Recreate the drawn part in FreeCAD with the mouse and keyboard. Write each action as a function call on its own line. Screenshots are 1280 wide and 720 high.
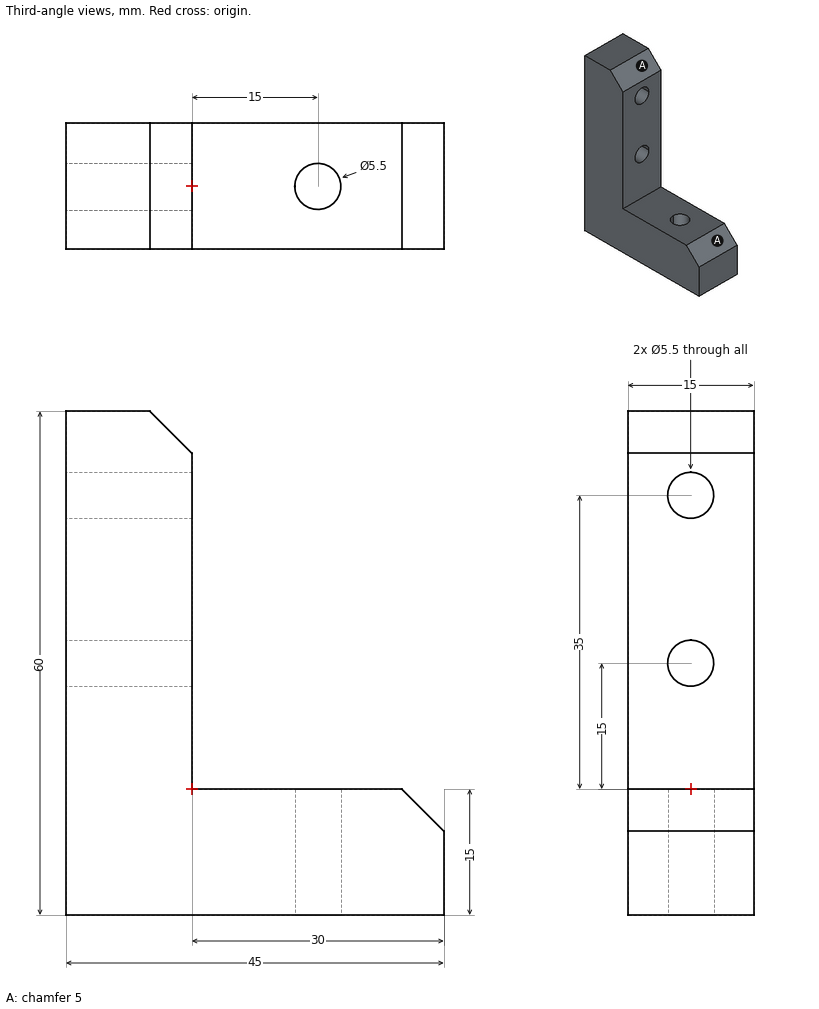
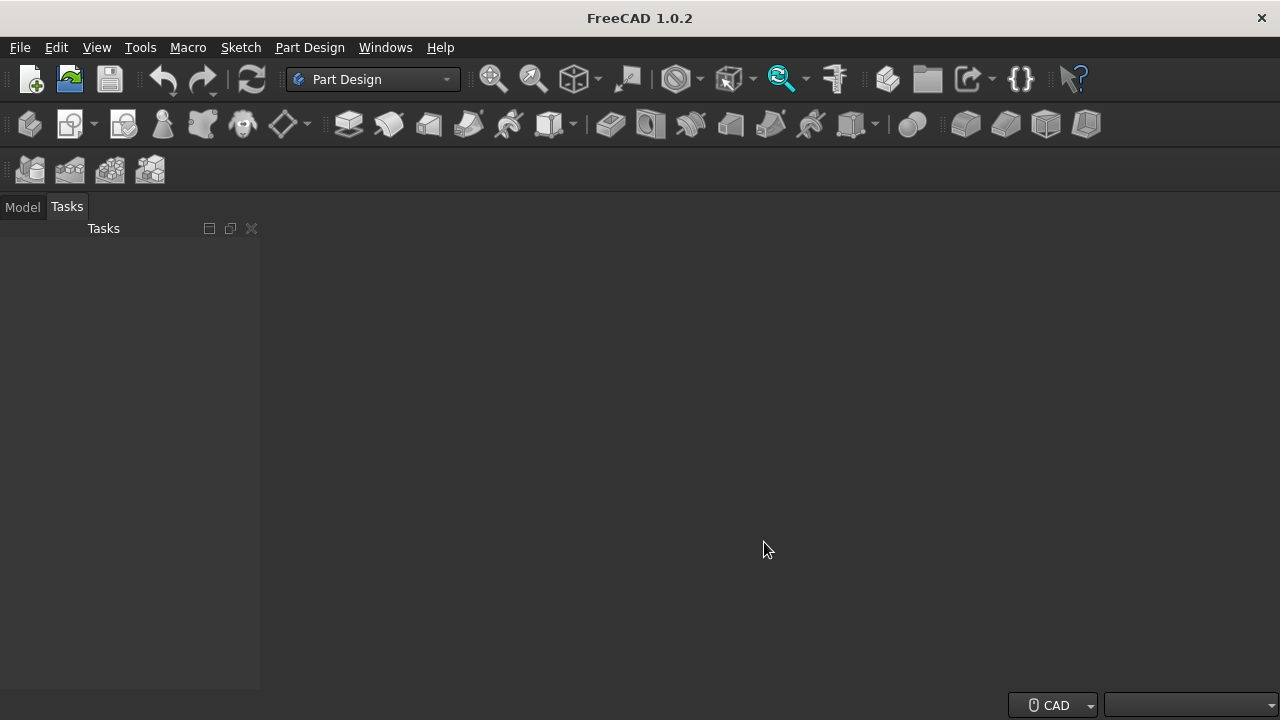
key(ctrl+n)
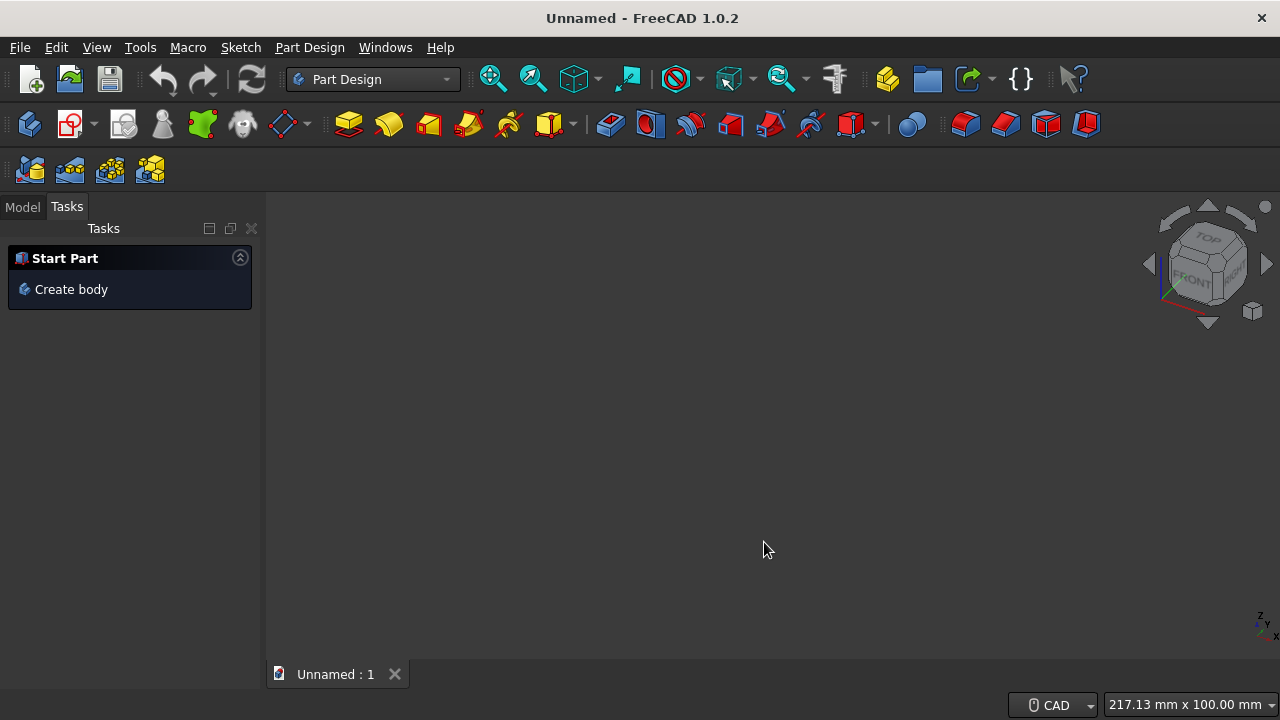
click(70, 124)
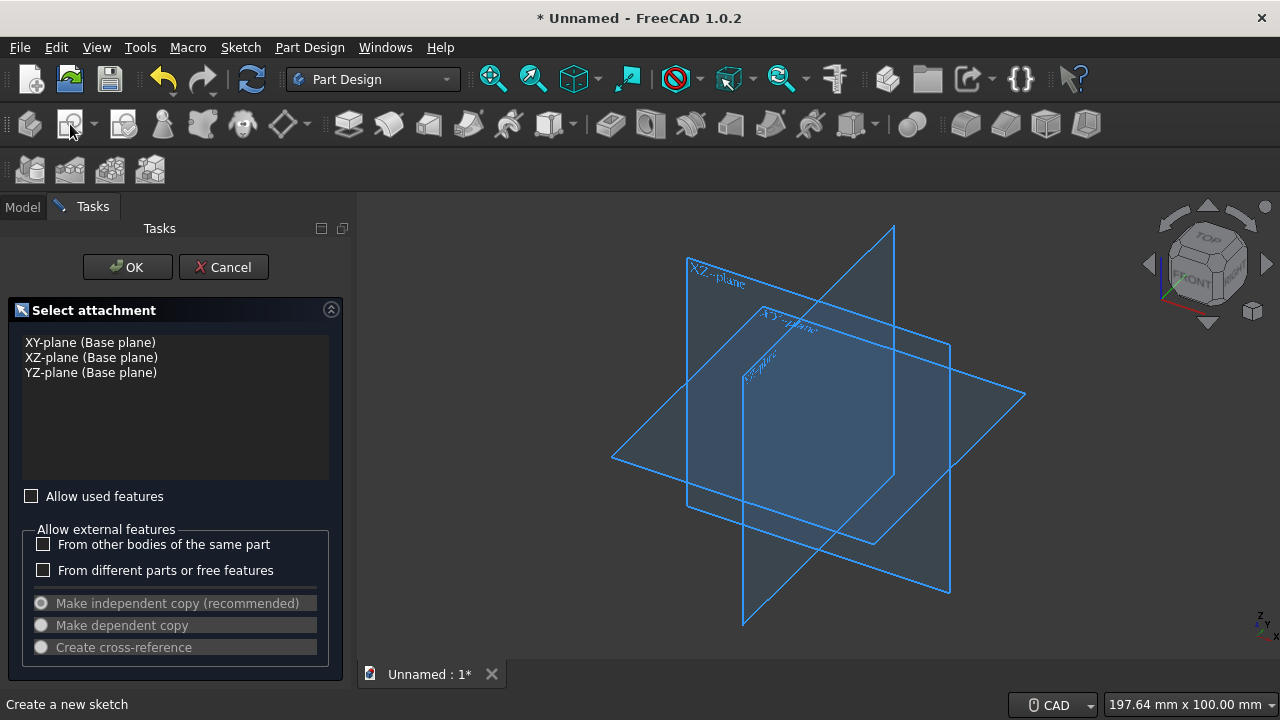
click(82, 358)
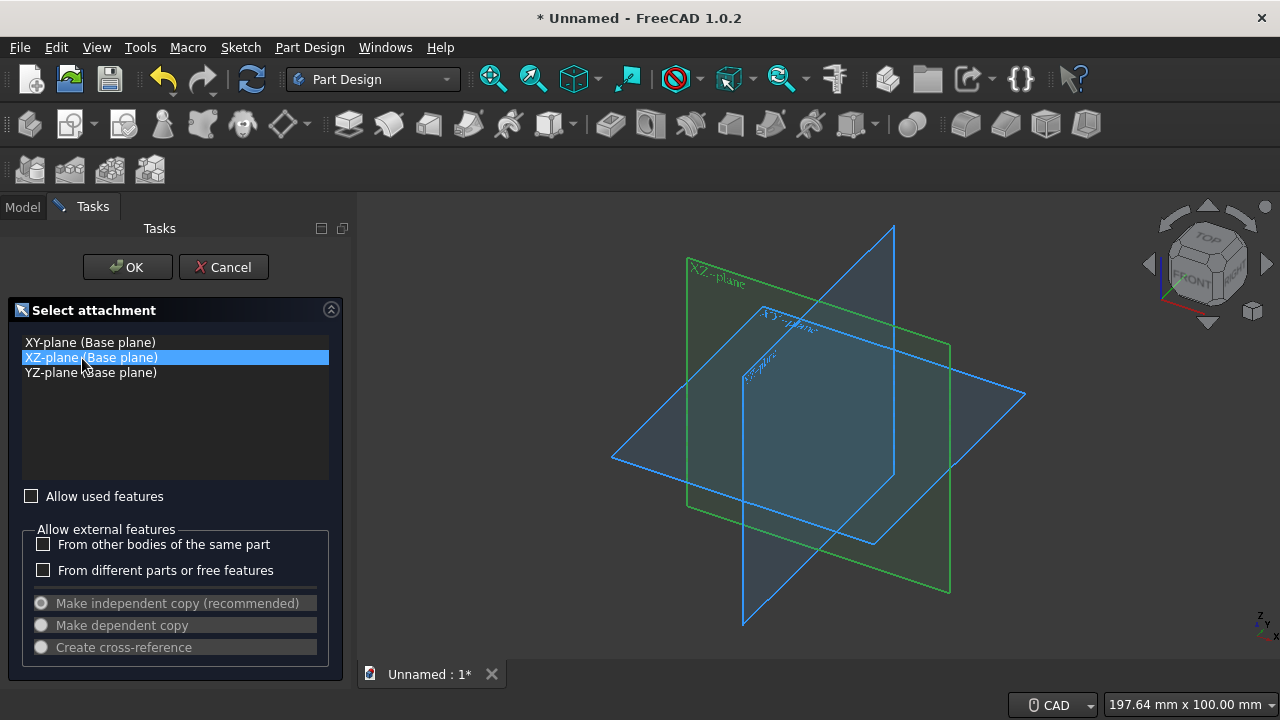
click(128, 267)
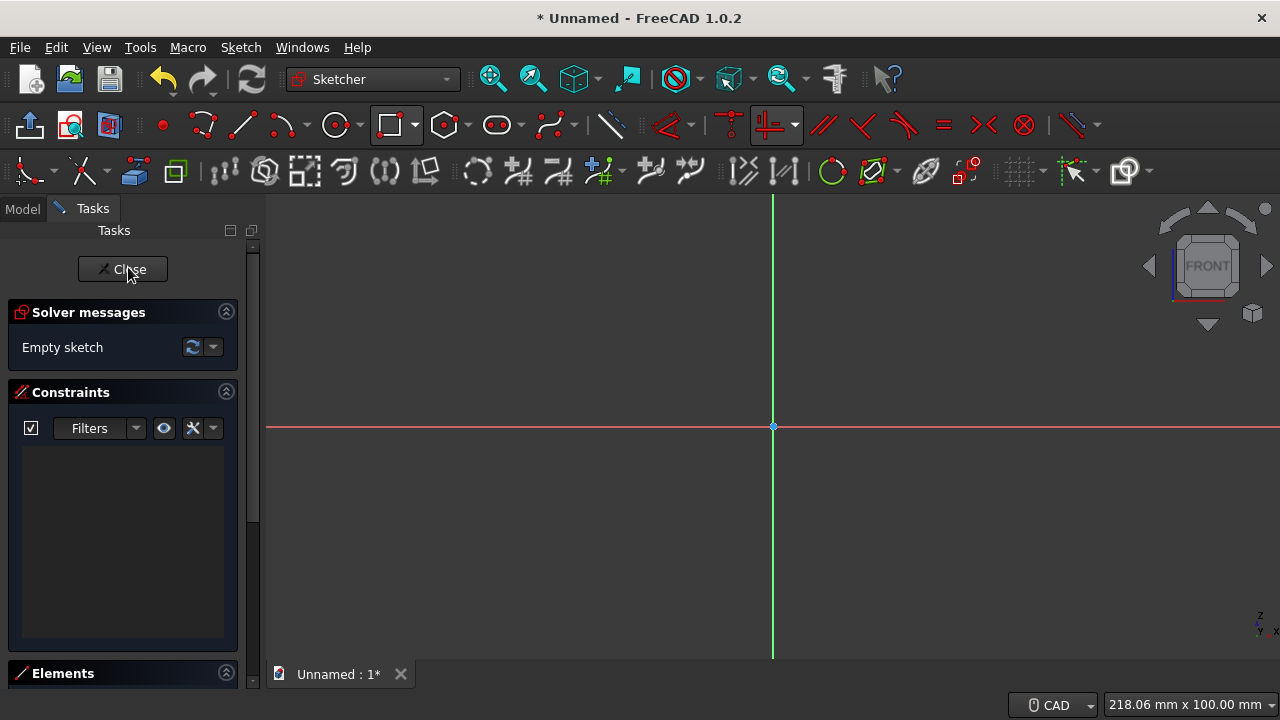
scroll(294, 631, down, 1)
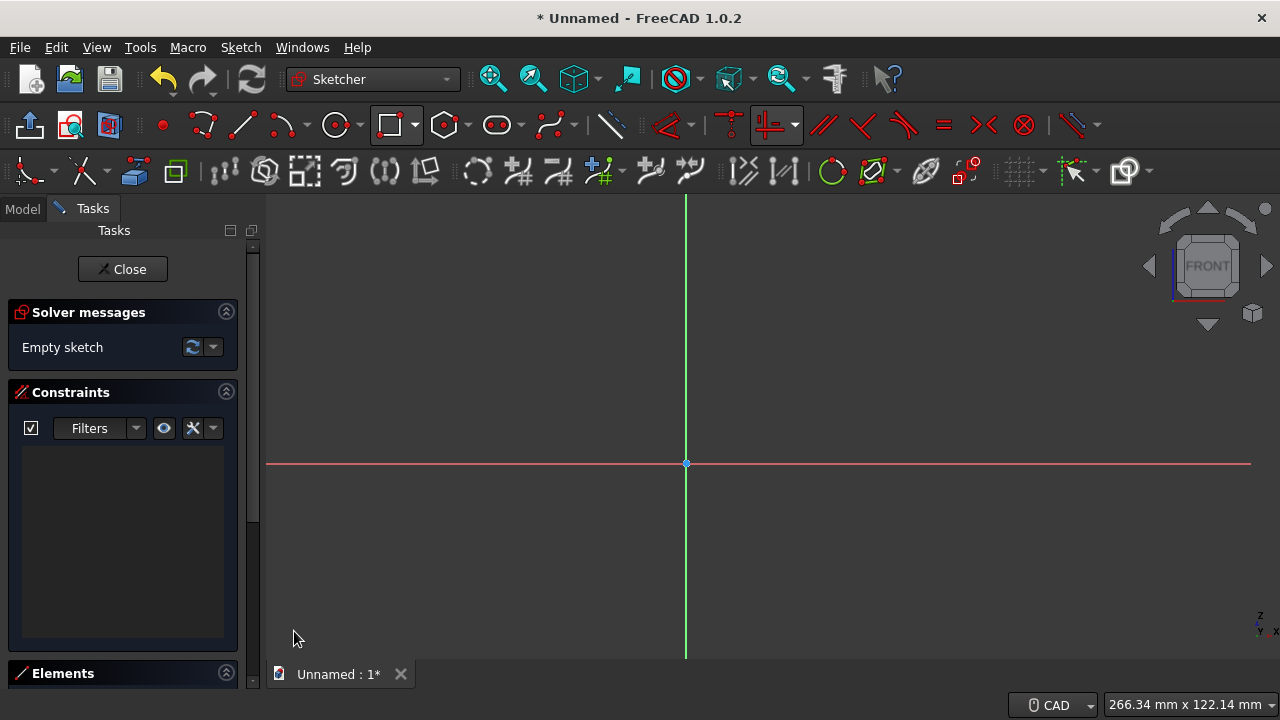
key(g)
key(m)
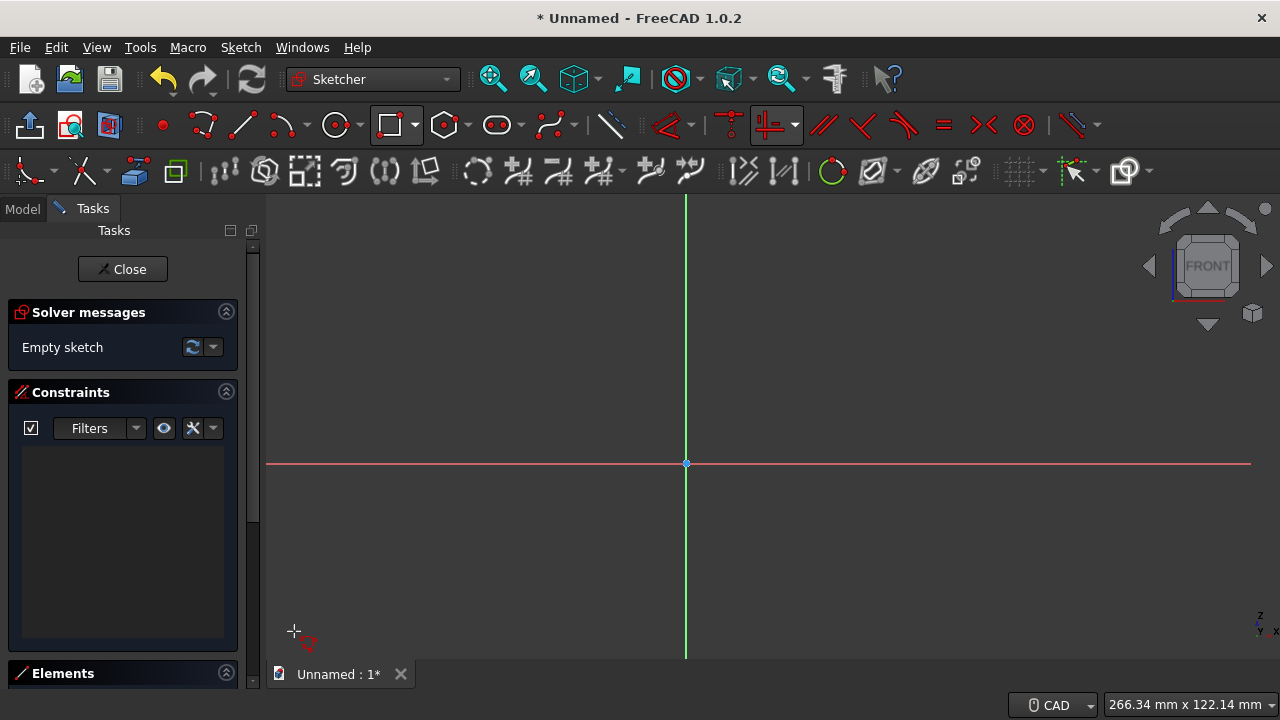
click(686, 464)
click(800, 455)
click(800, 521)
click(629, 521)
click(629, 292)
click(695, 292)
click(686, 464)
key(Escape)
key(Escape)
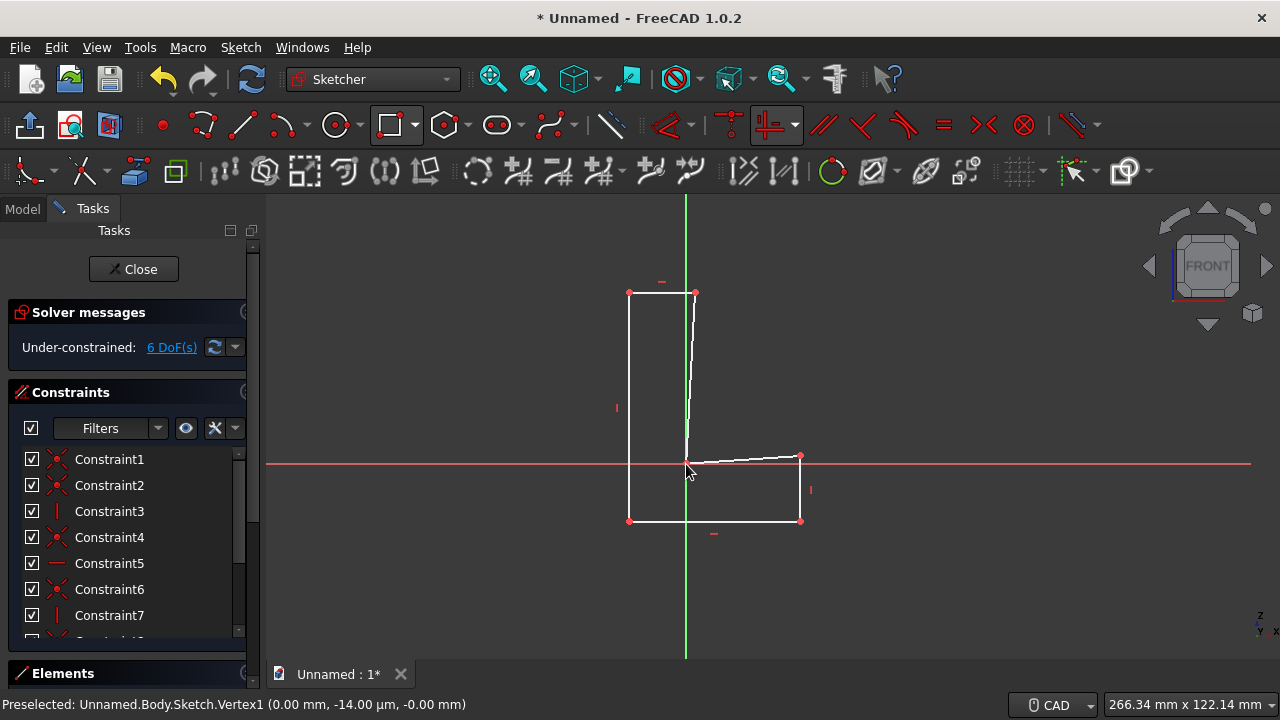
click(720, 461)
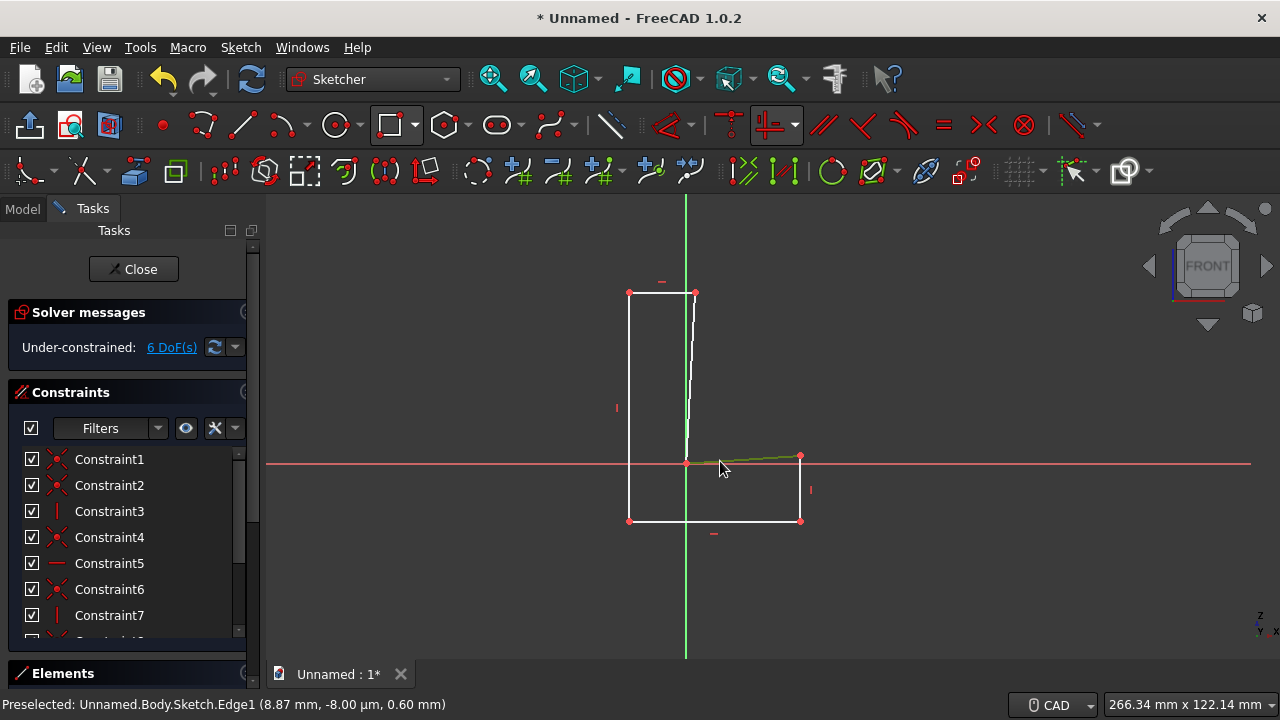
click(798, 126)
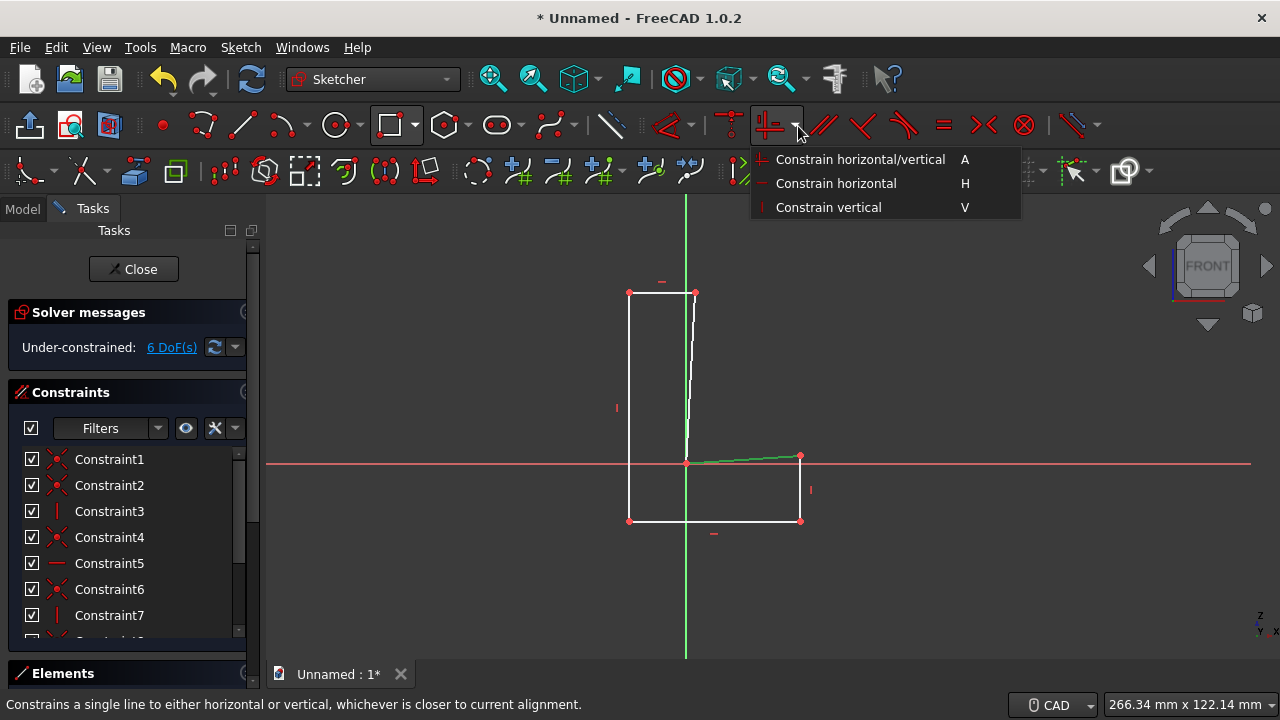
click(886, 183)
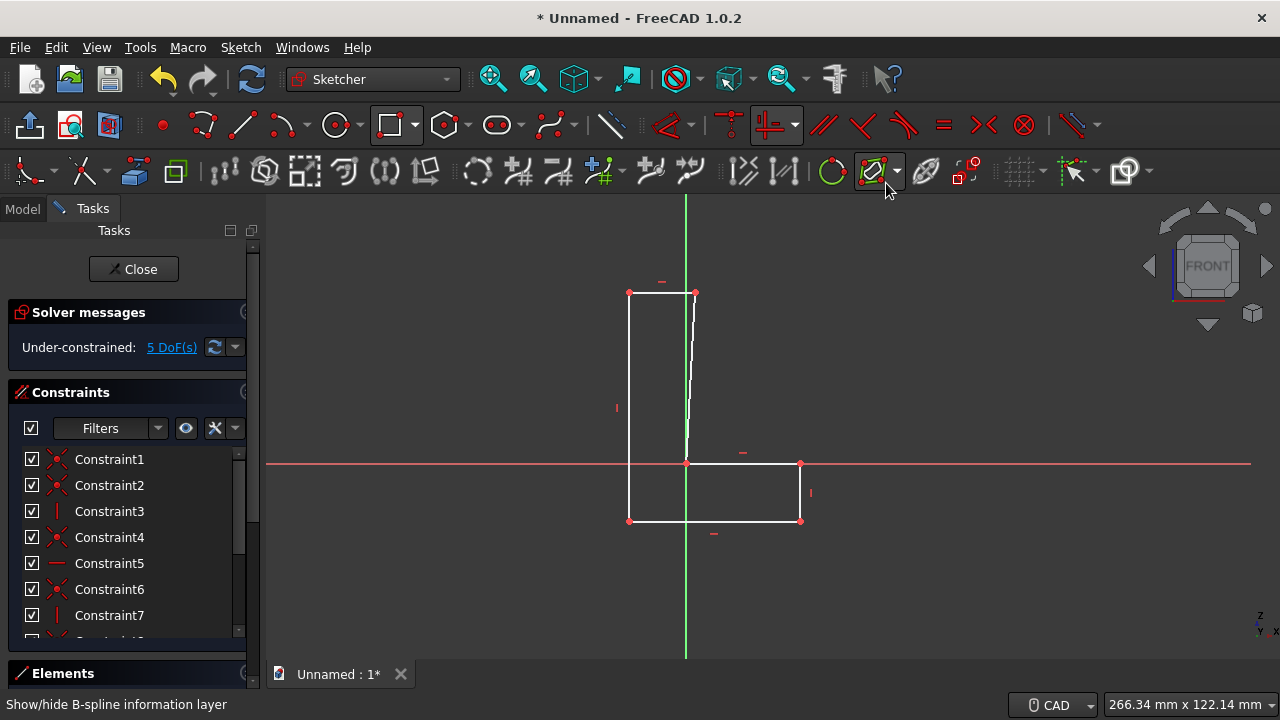
click(689, 413)